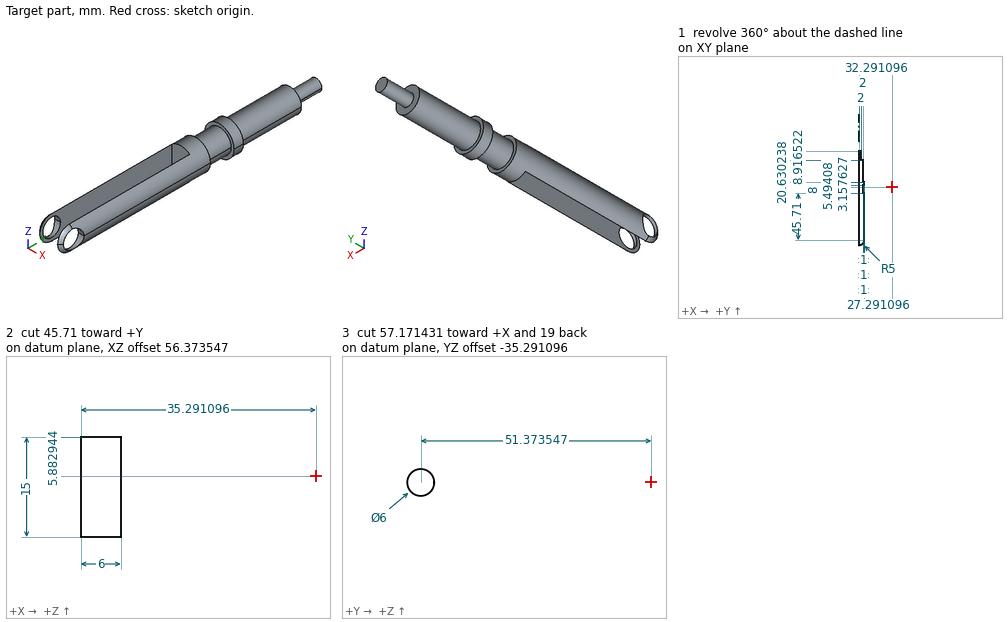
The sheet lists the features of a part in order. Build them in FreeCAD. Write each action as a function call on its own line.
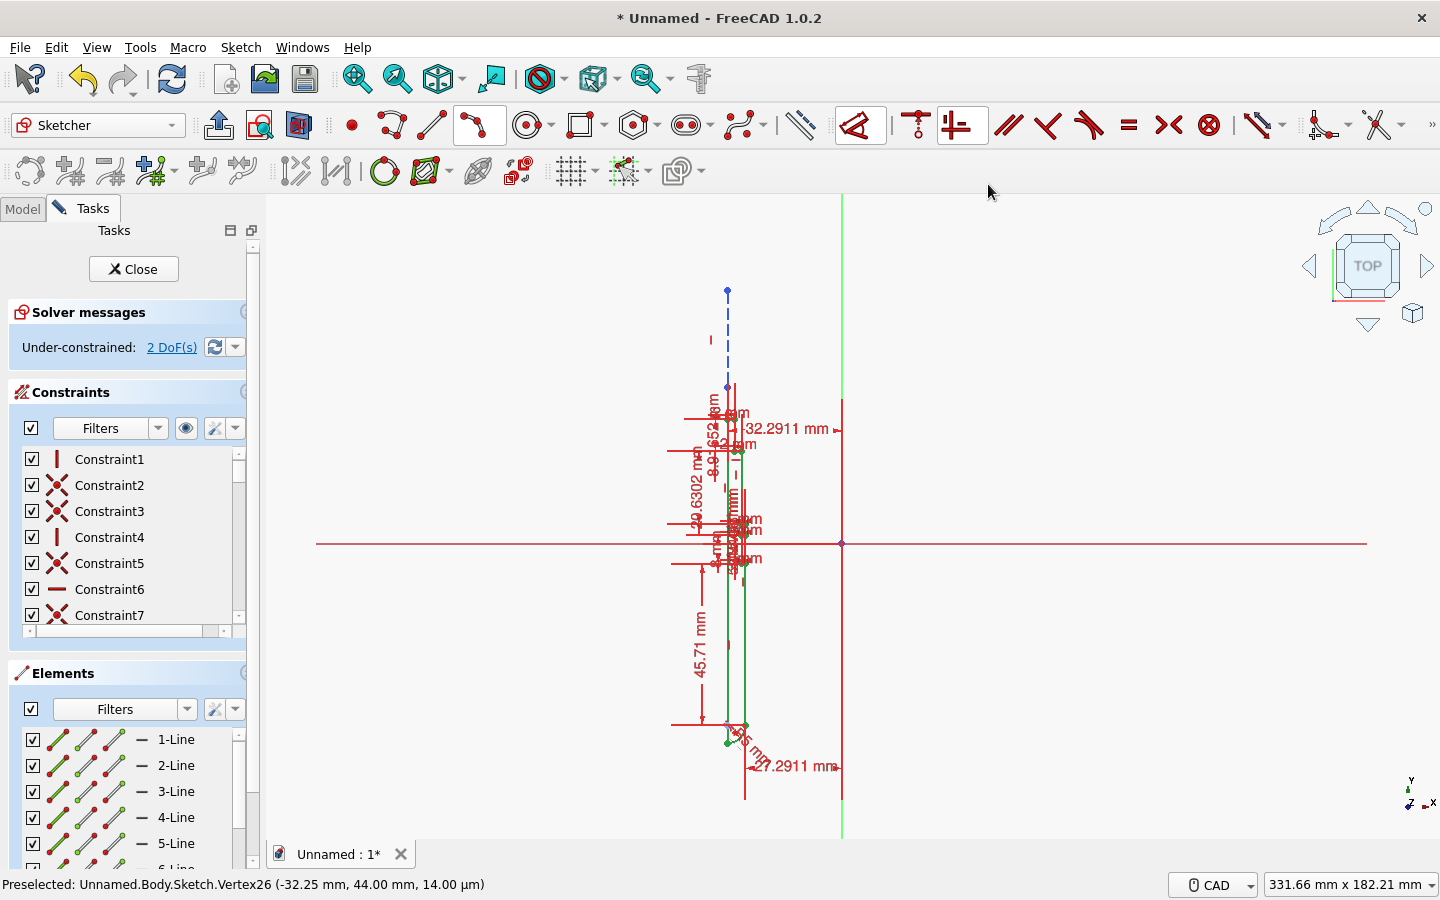
click(134, 269)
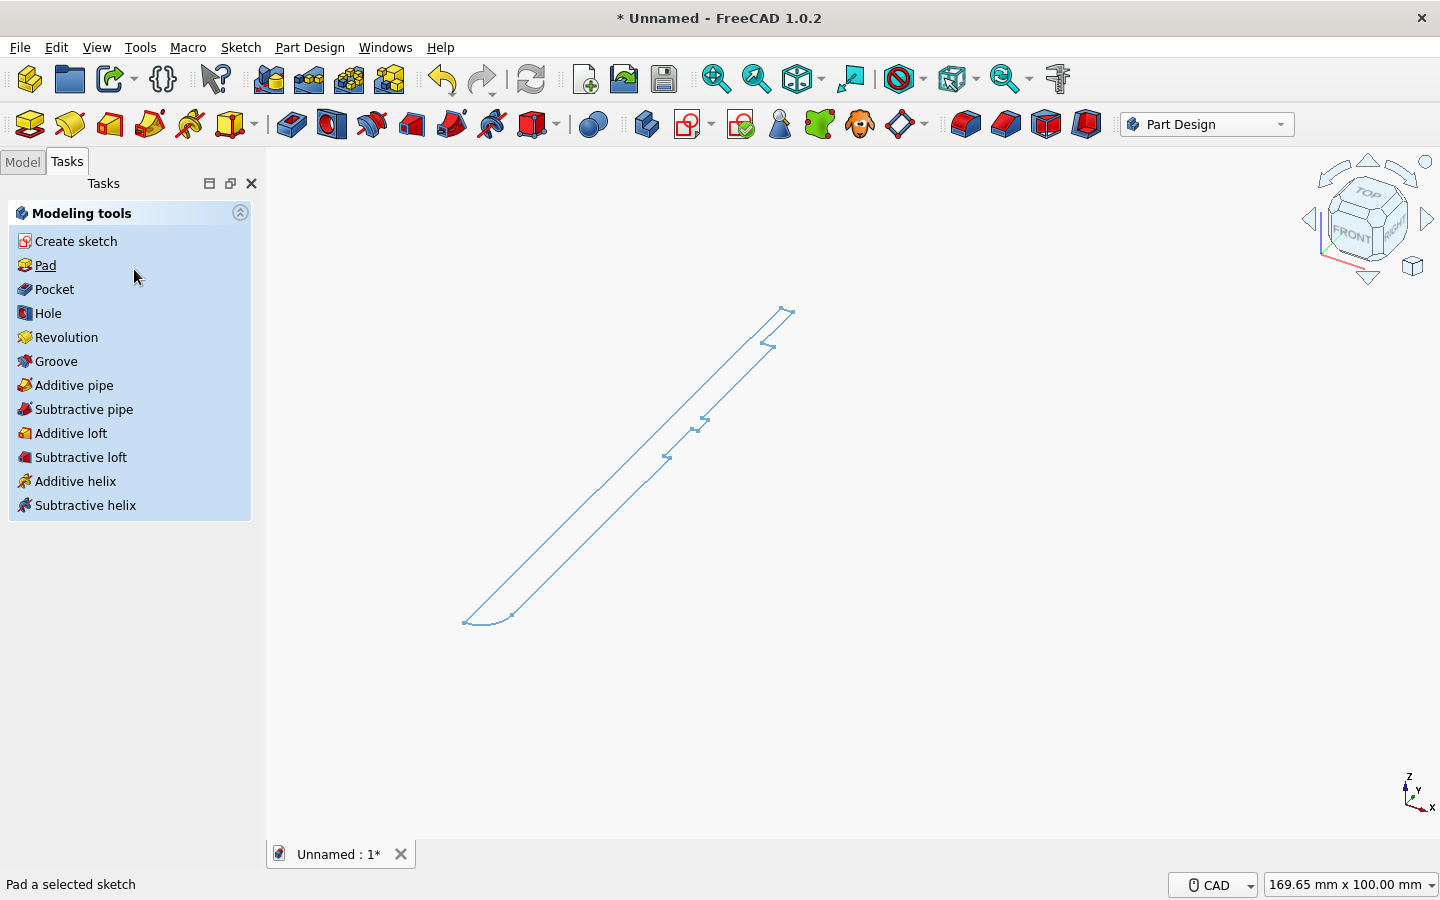
click(70, 124)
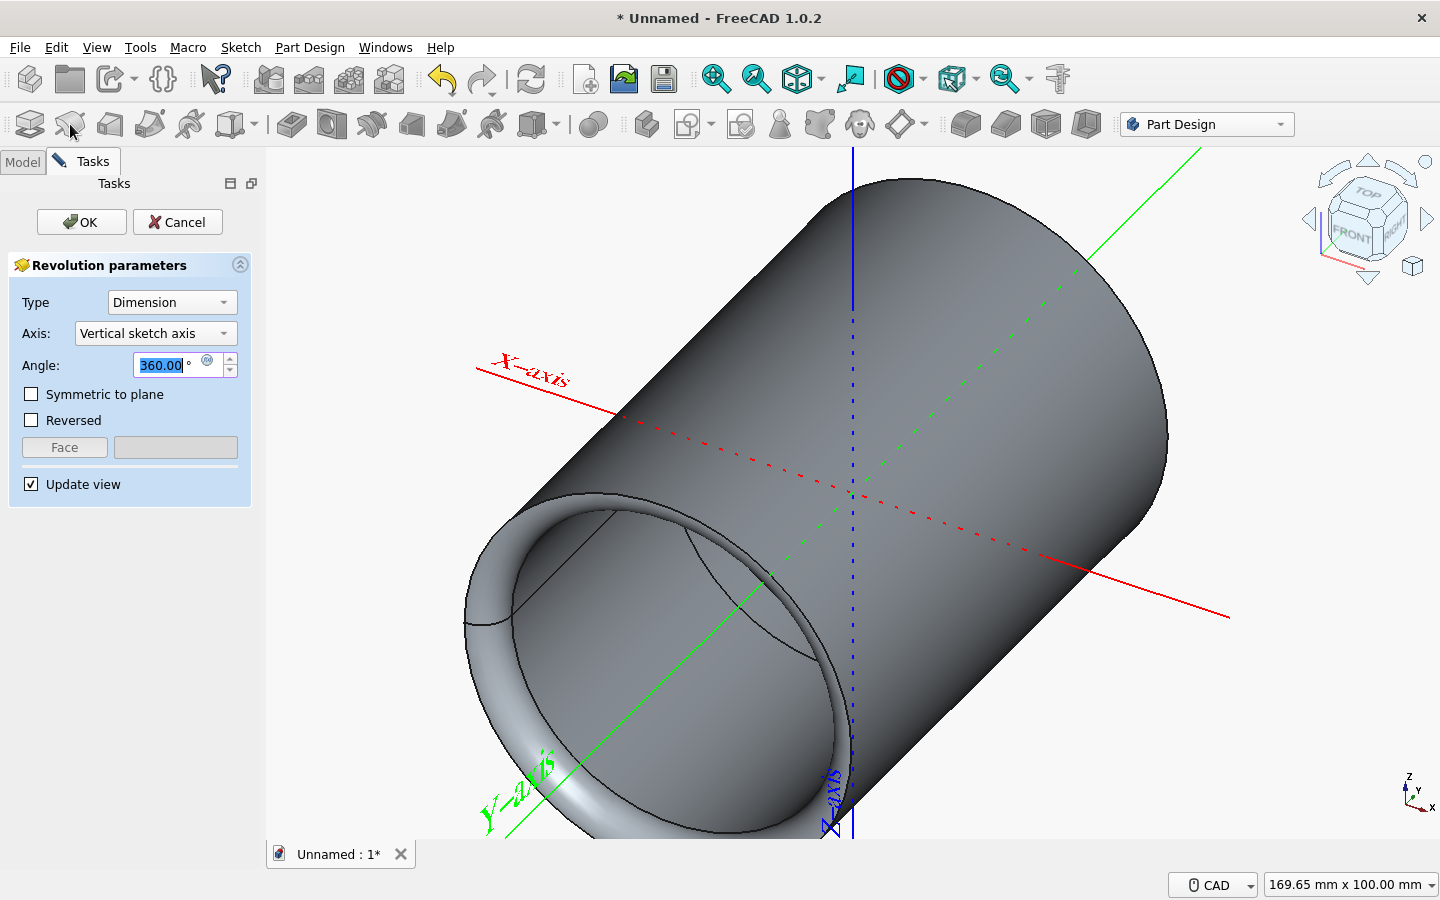
click(156, 334)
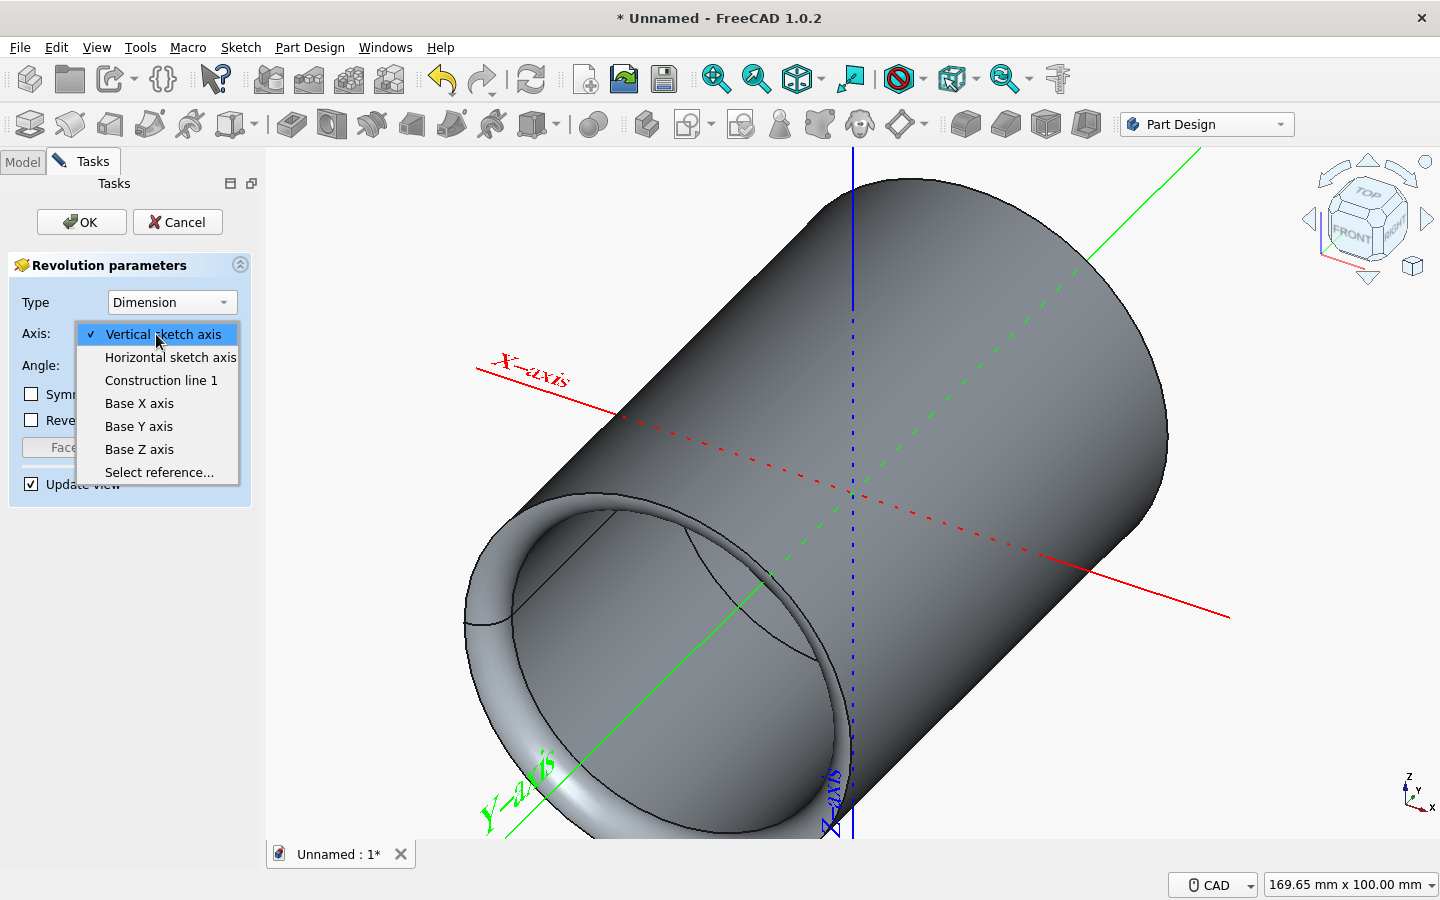
click(156, 380)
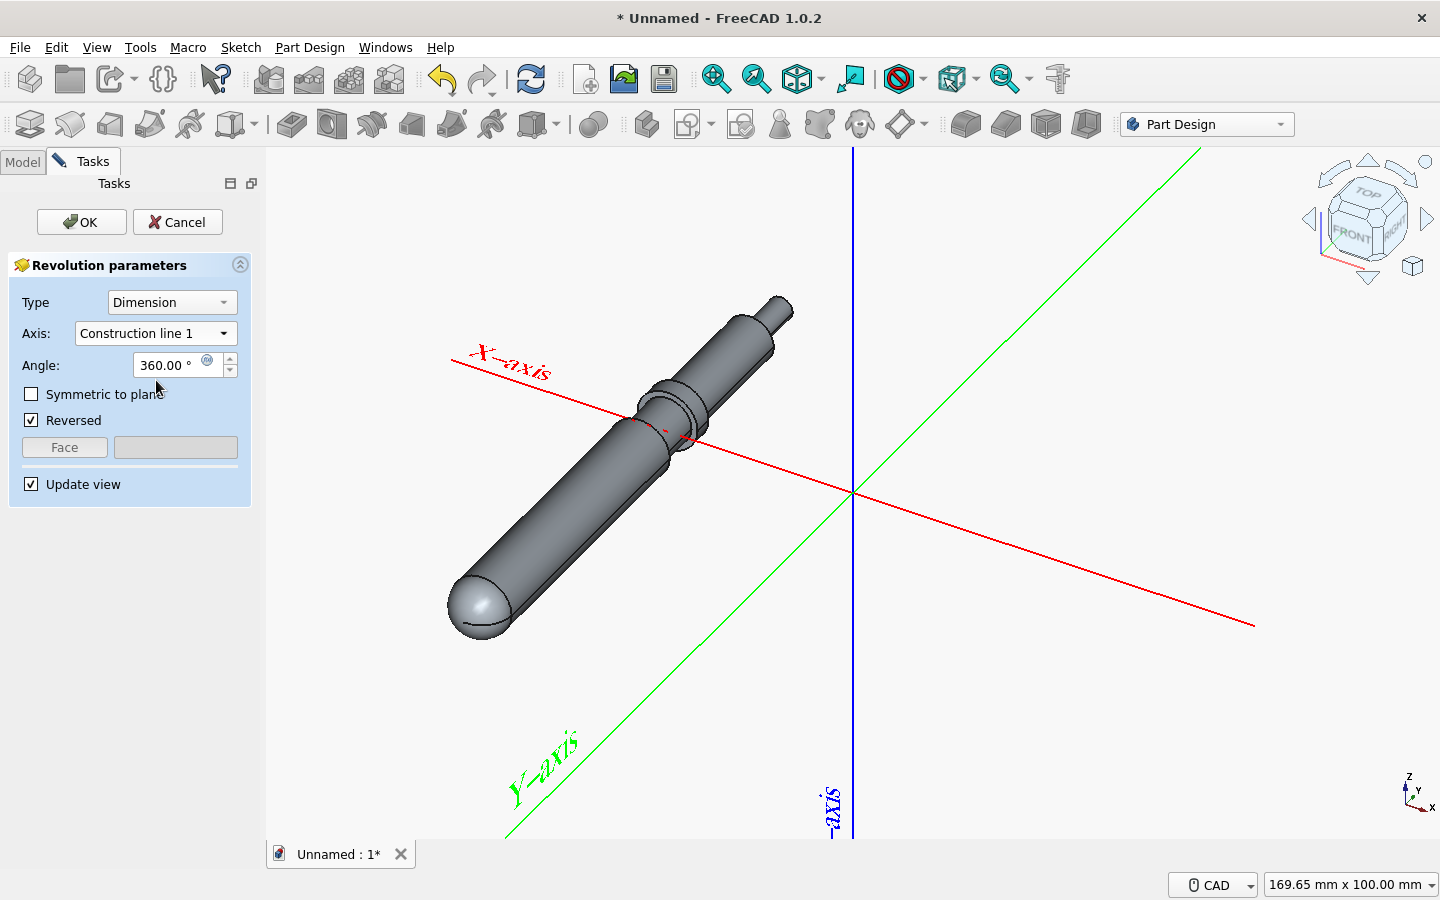
click(82, 222)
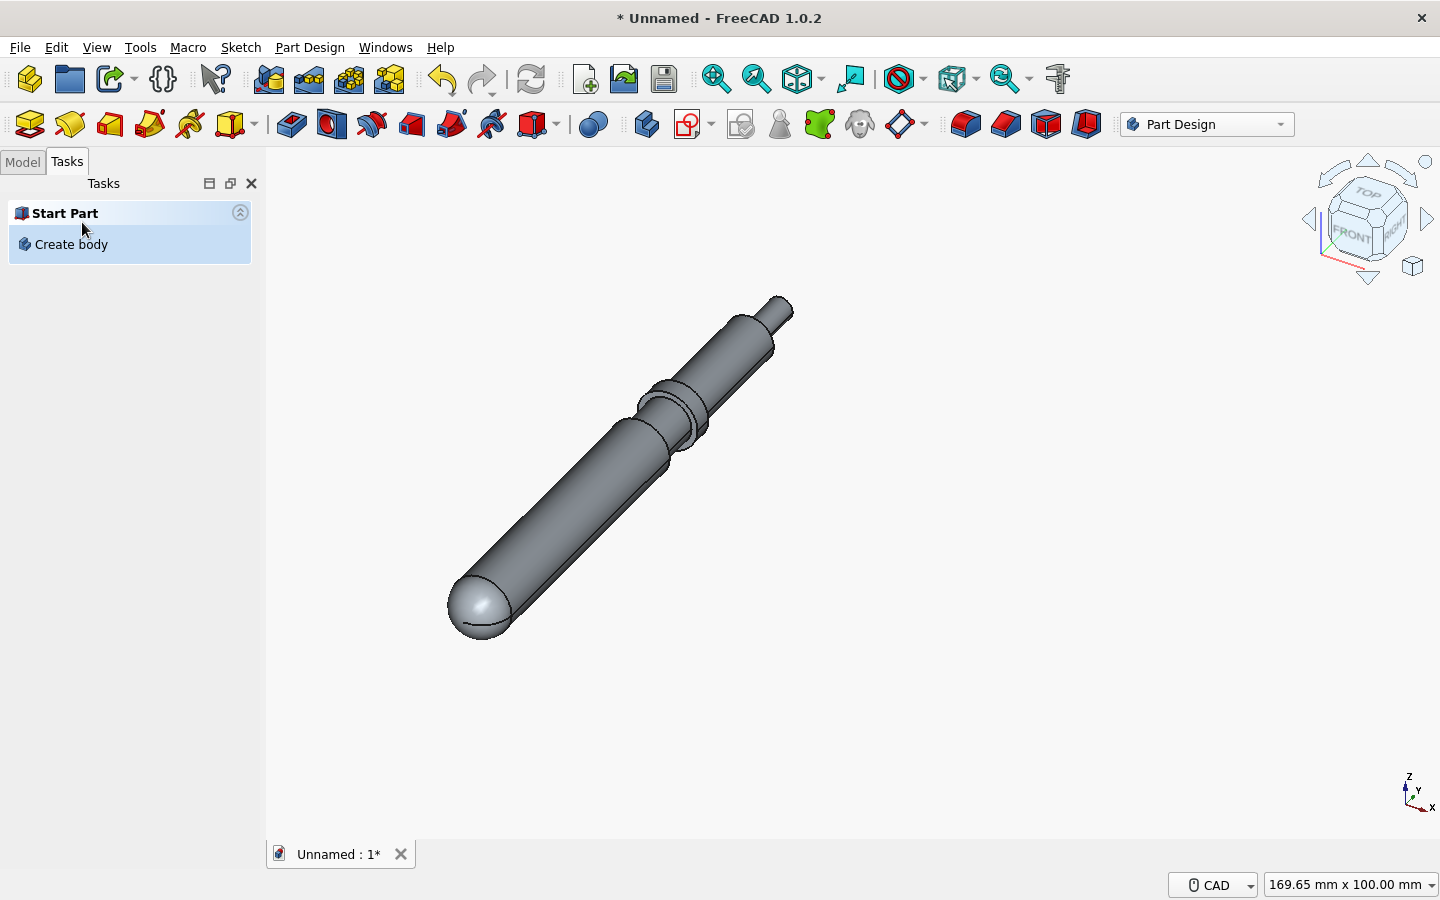
click(23, 161)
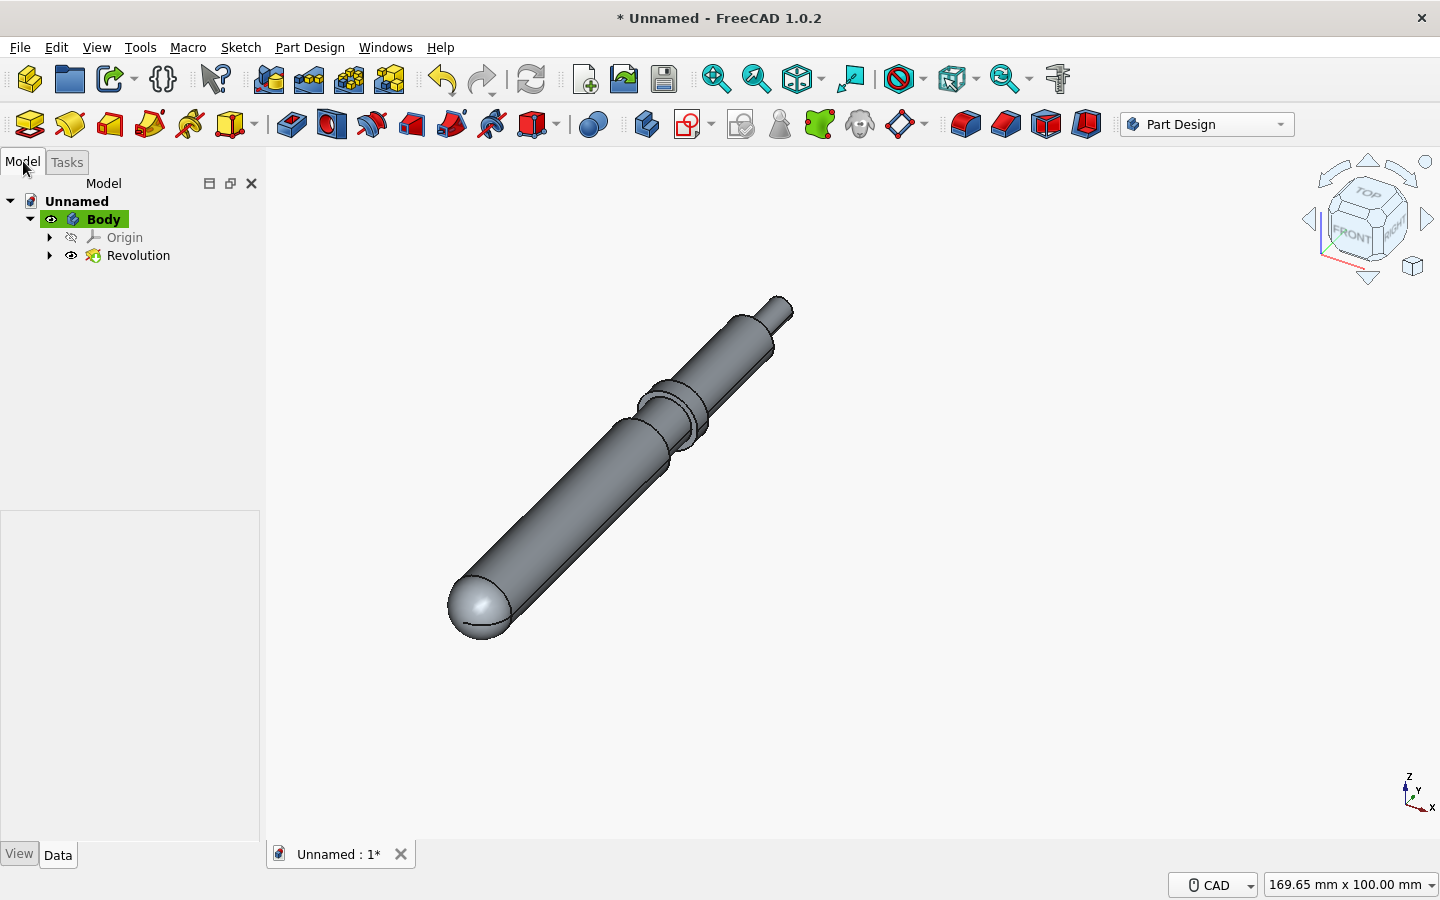
click(50, 237)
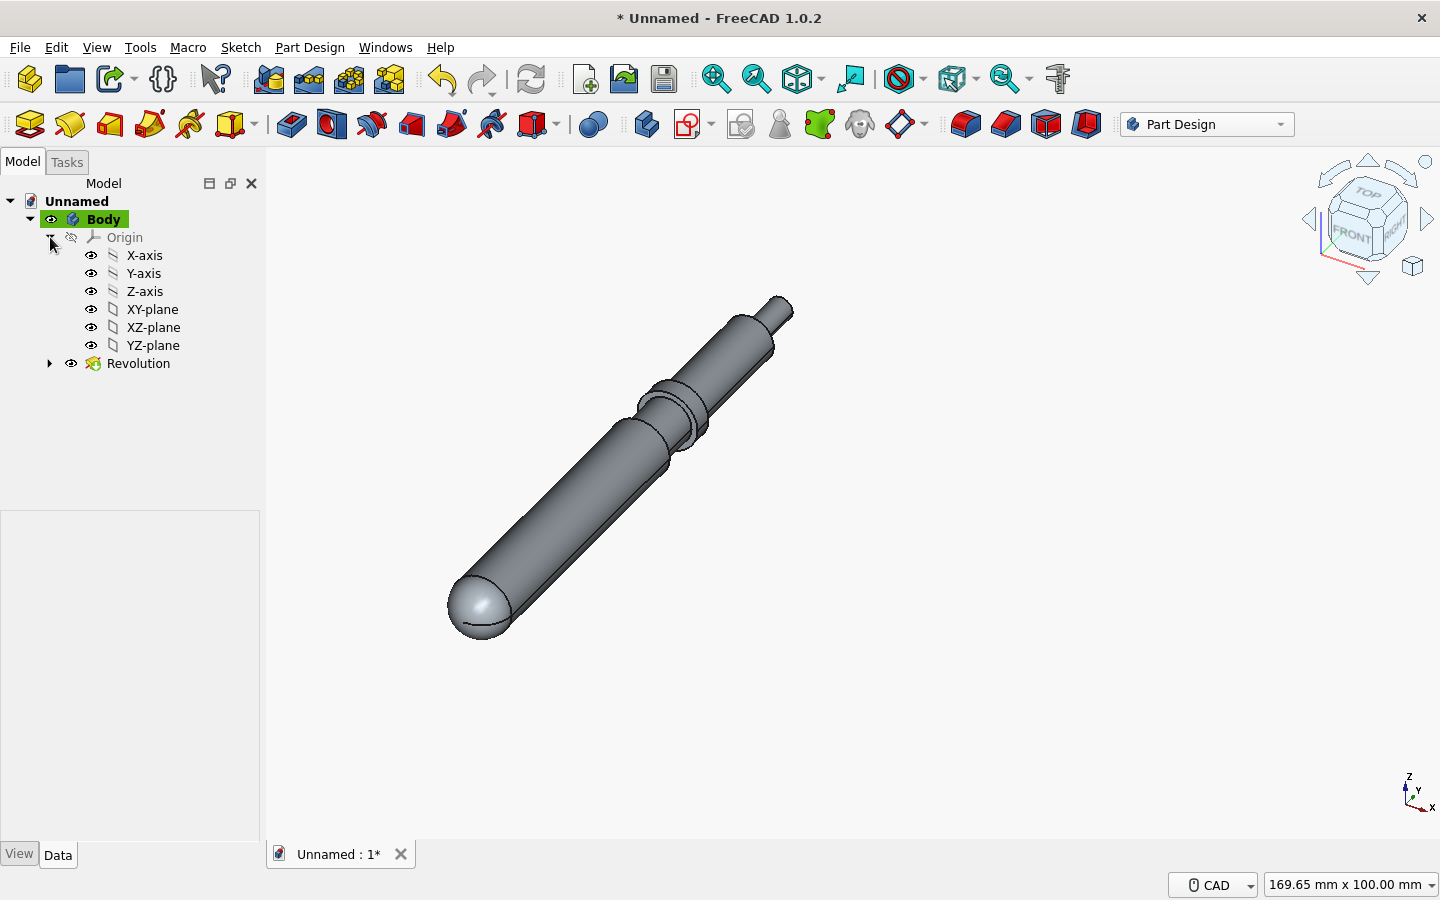
click(136, 327)